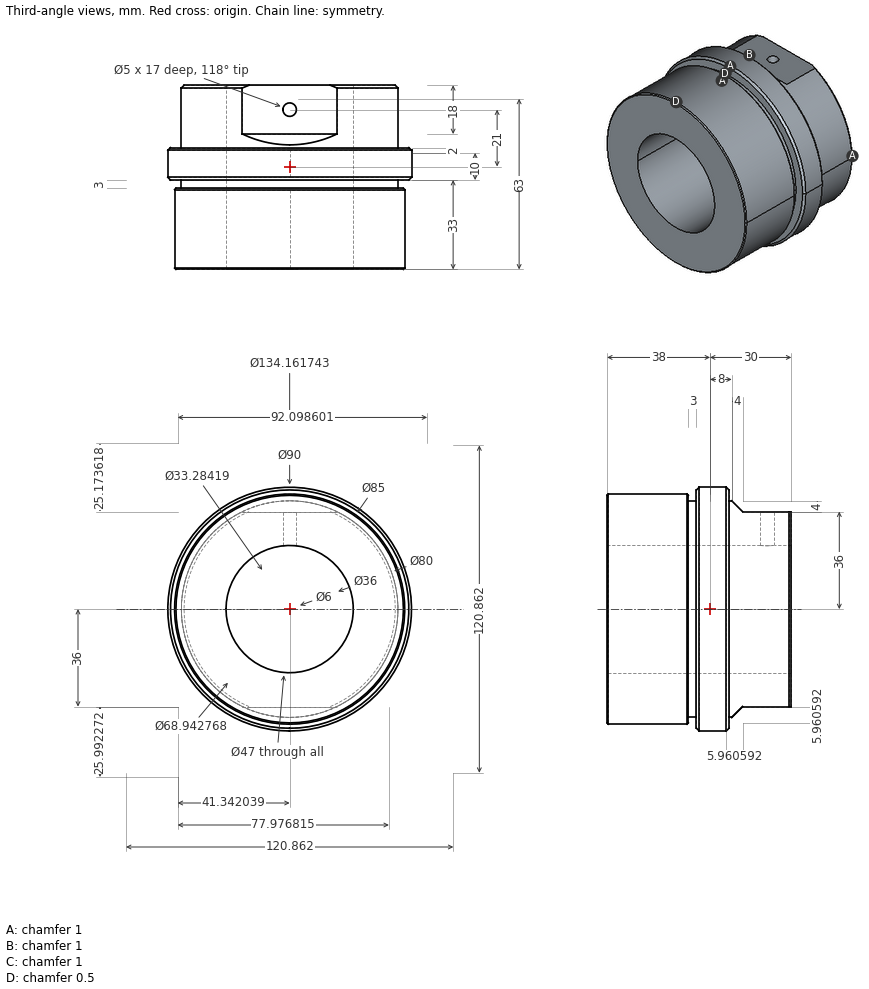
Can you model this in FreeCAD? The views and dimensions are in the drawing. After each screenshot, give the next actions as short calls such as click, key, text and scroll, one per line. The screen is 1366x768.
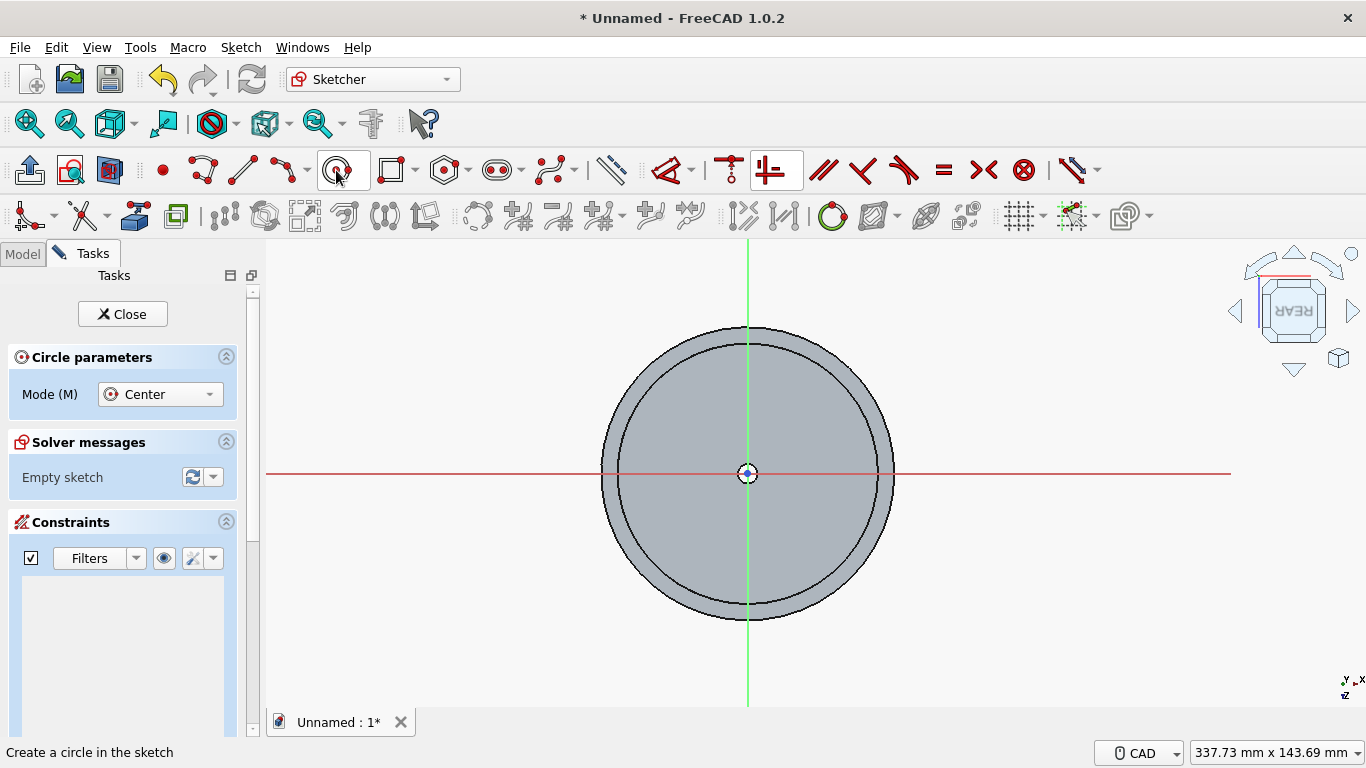
click(748, 474)
click(851, 370)
key(Escape)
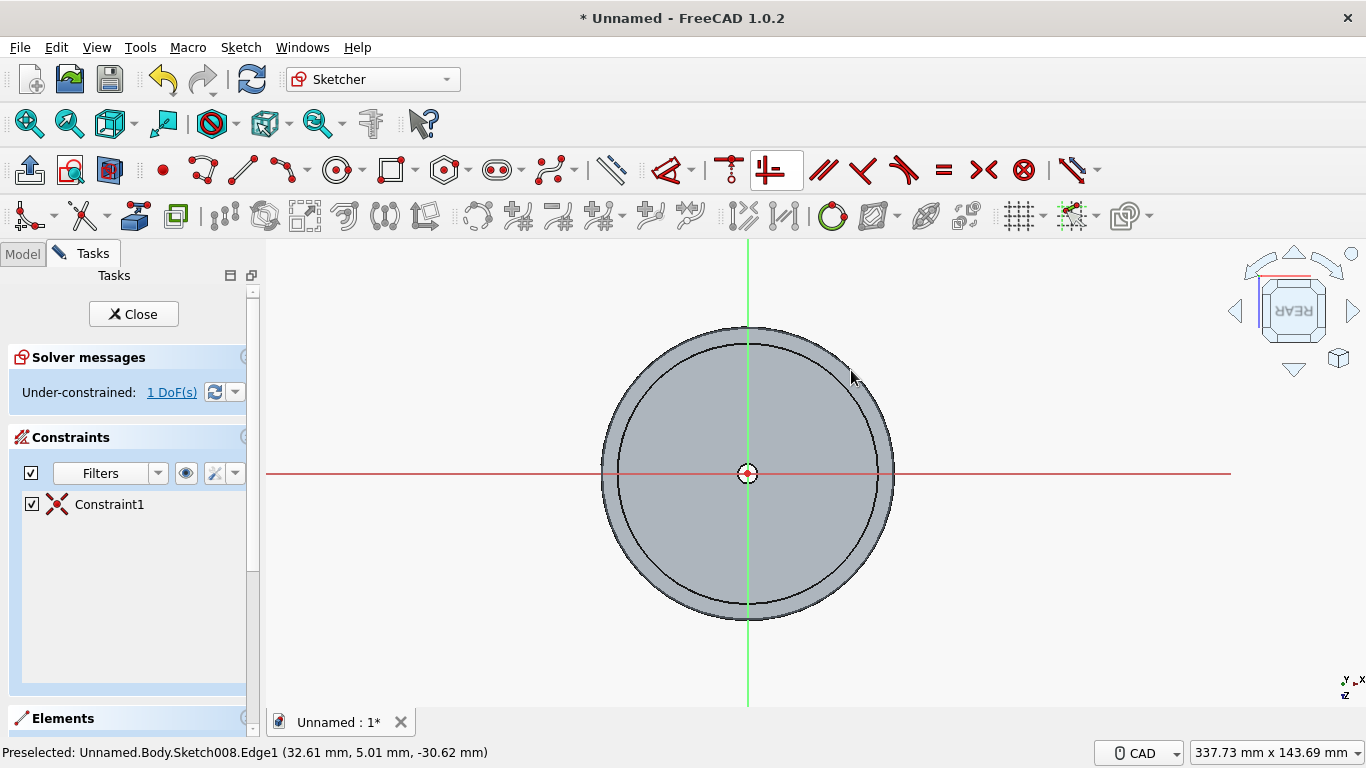
click(666, 170)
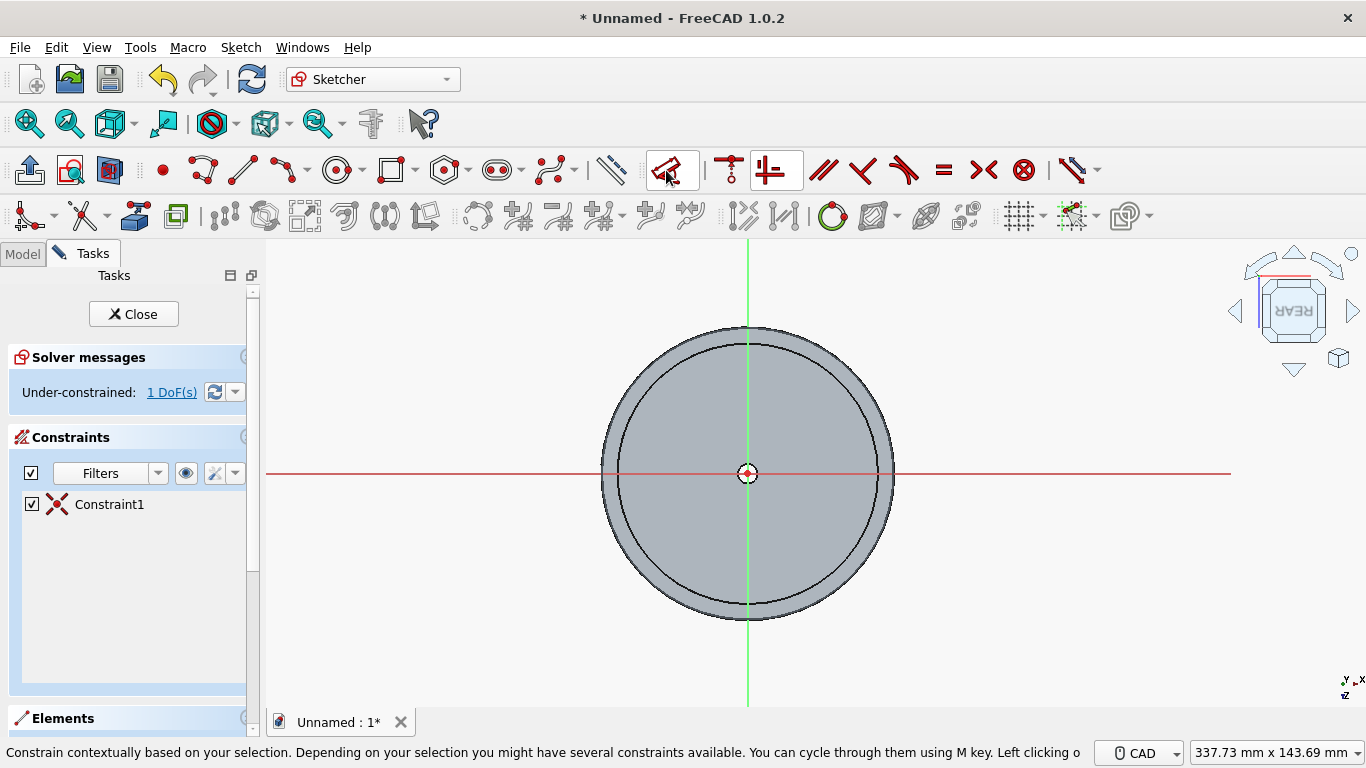
click(850, 370)
click(872, 347)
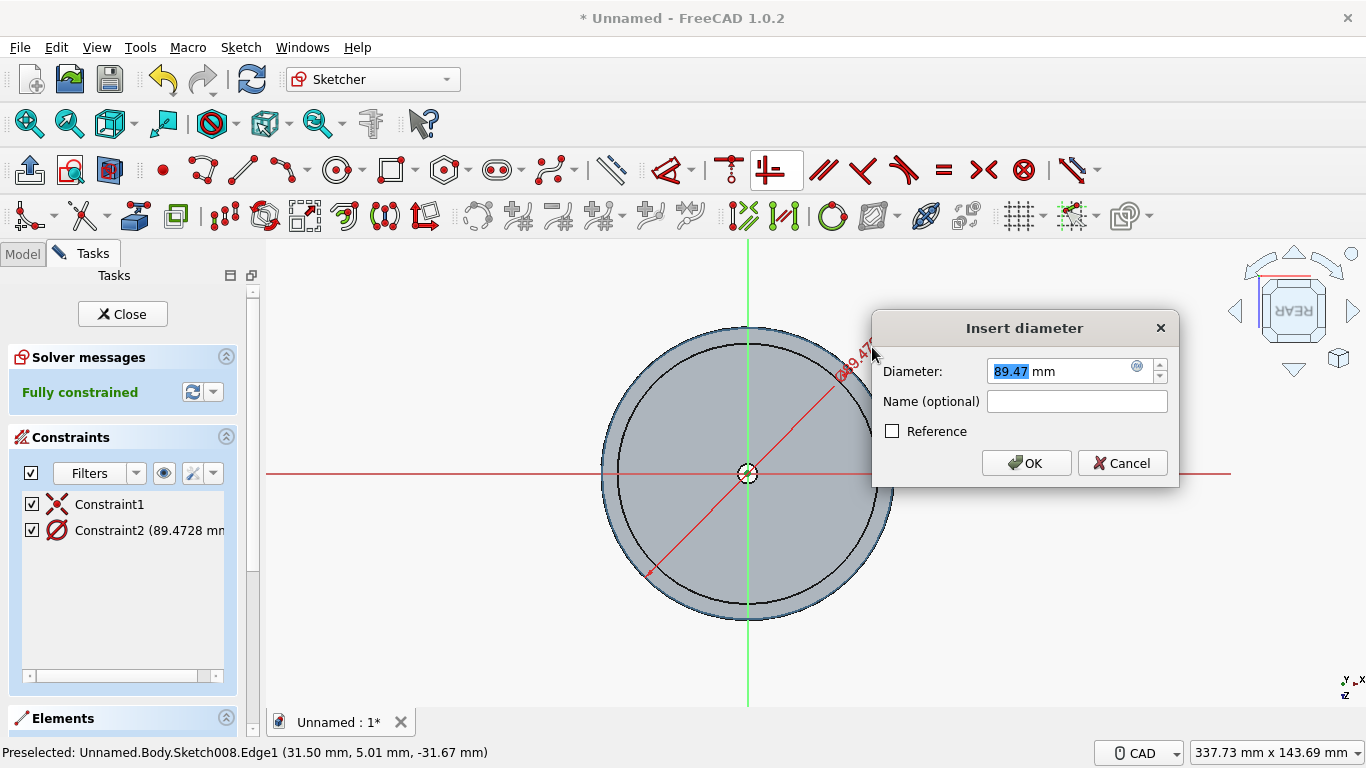
text(90)
key(Return)
key(Escape)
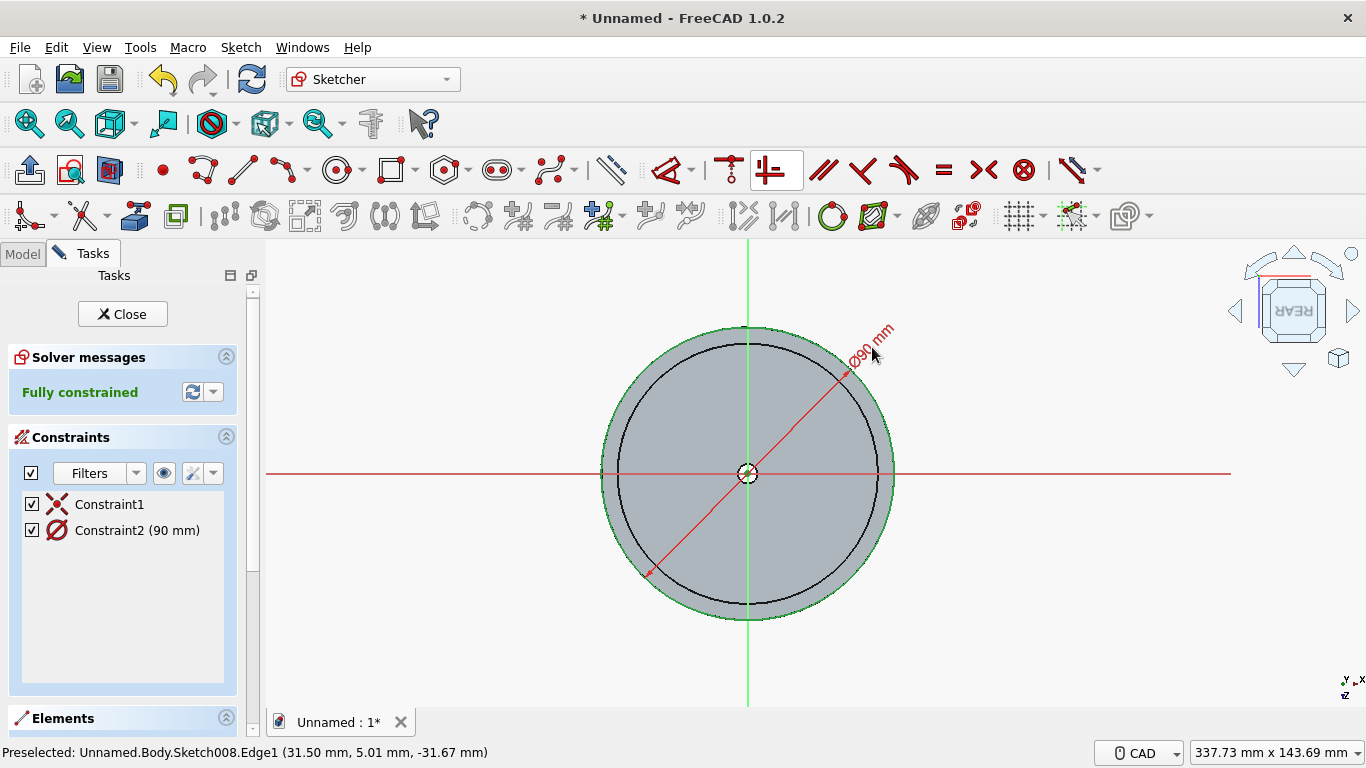
click(123, 314)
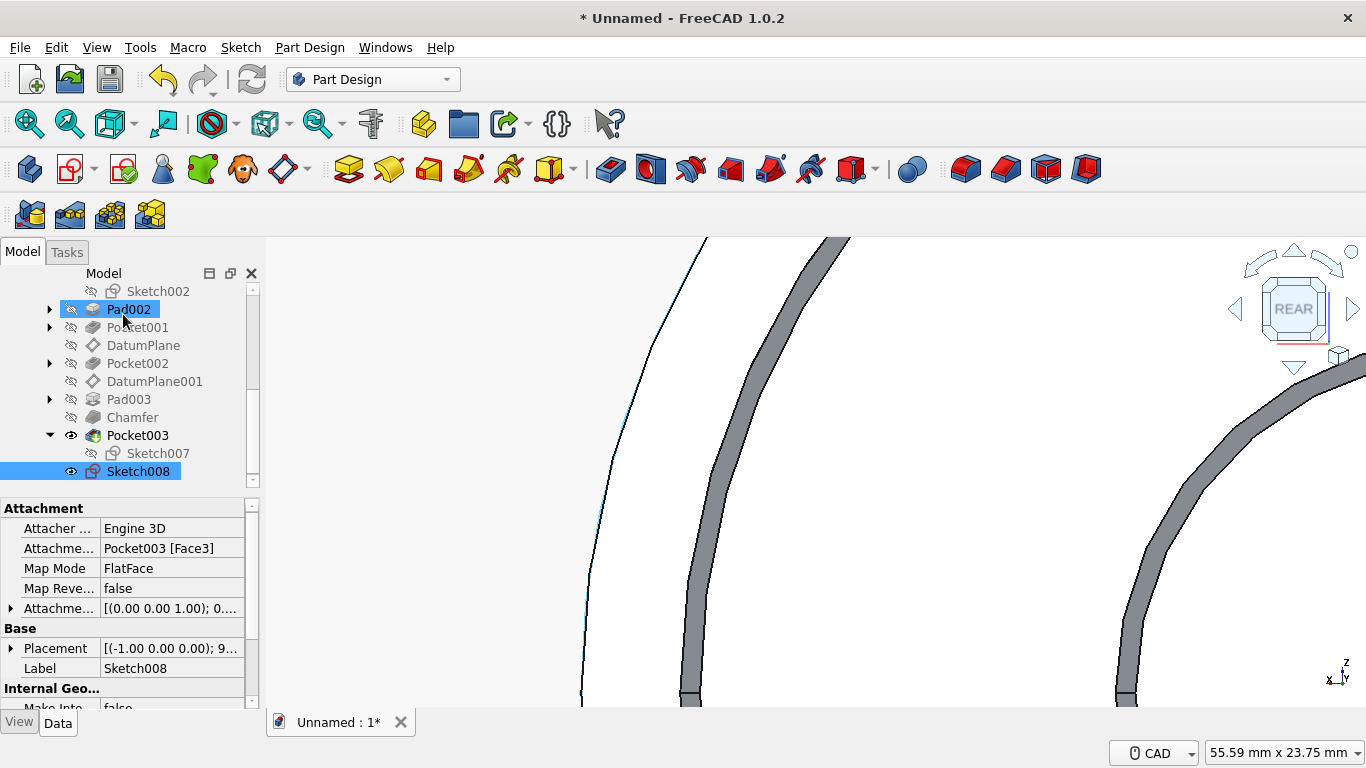
click(350, 170)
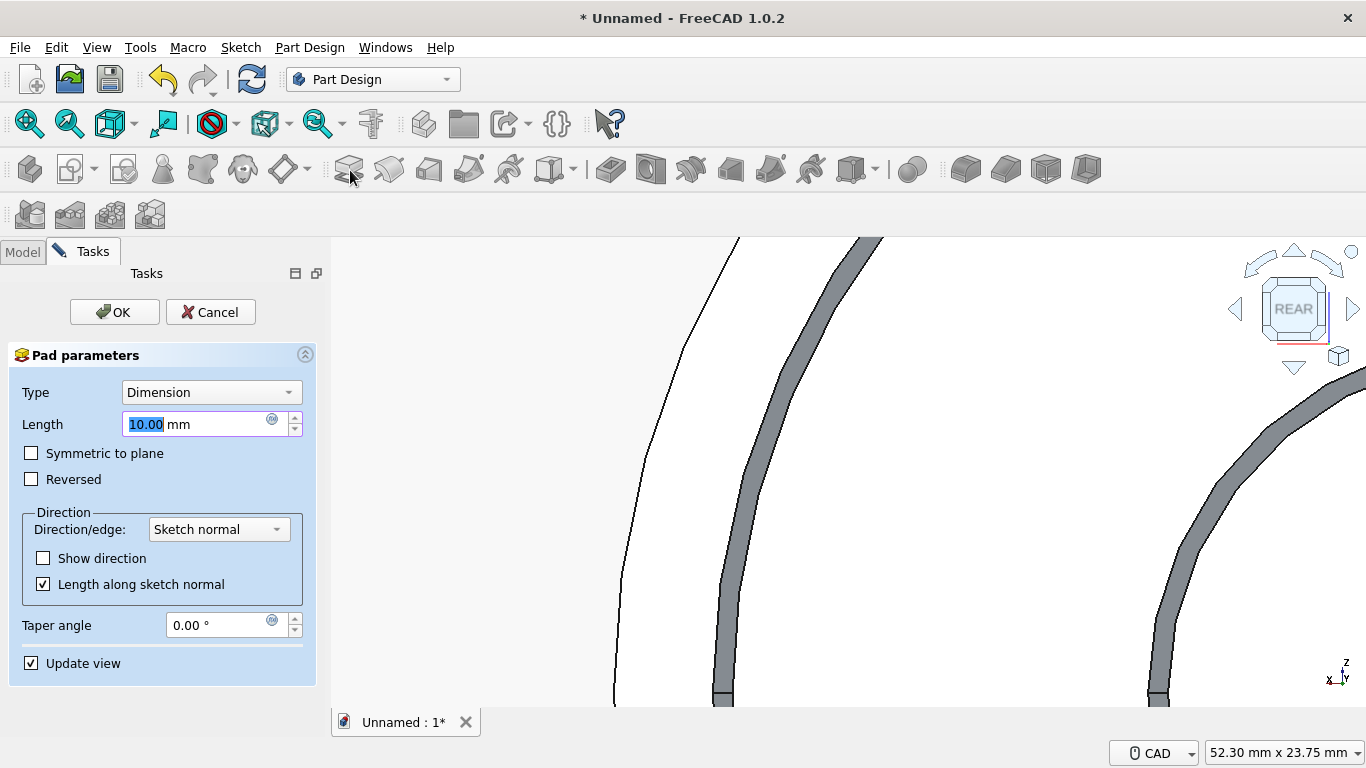
text(2)
key(Tab)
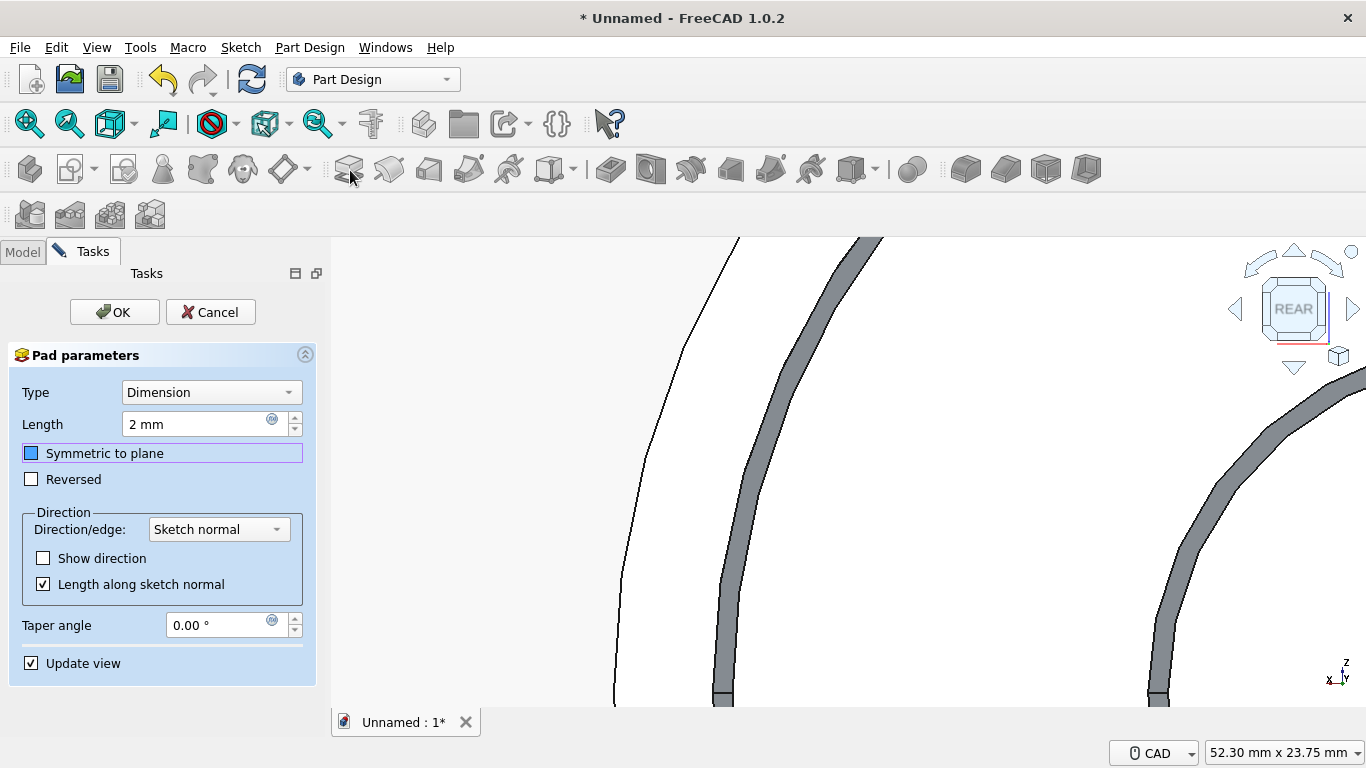
click(115, 312)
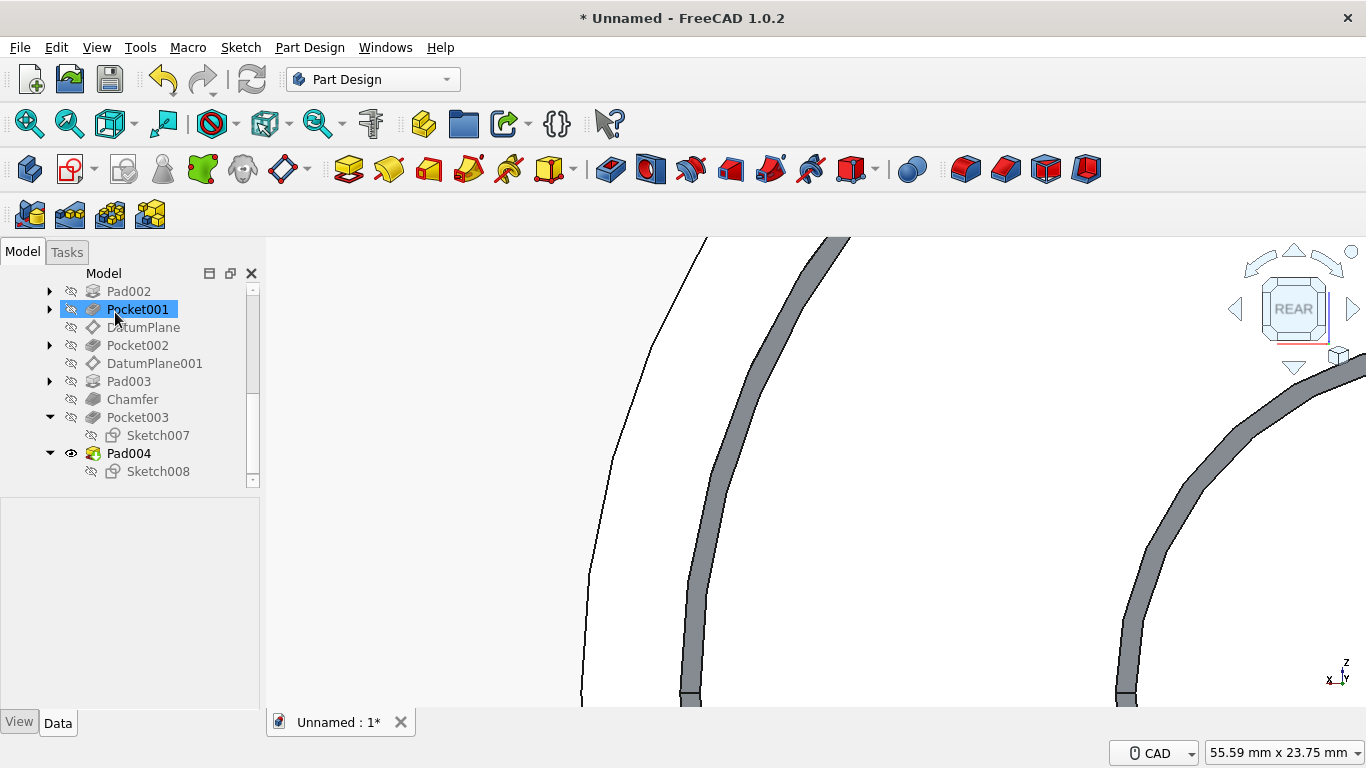
click(30, 124)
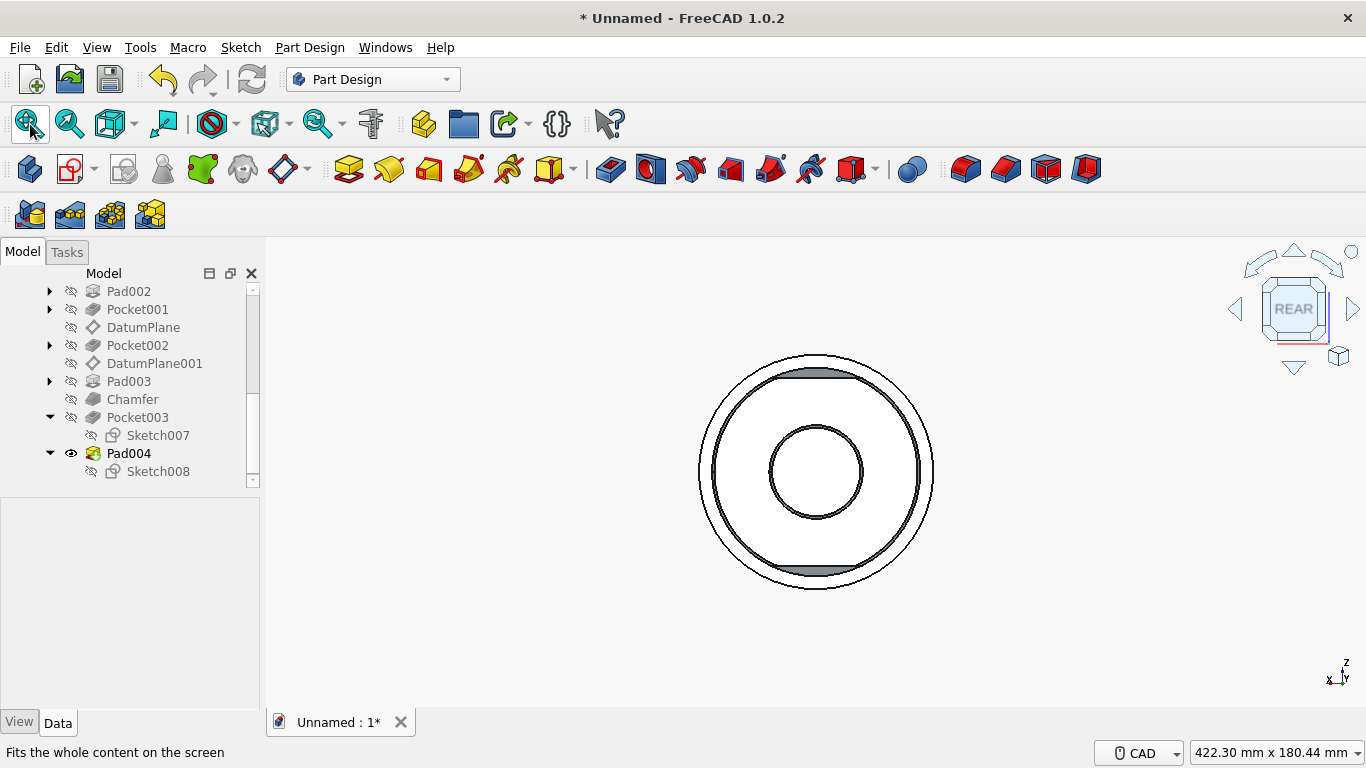
click(933, 471)